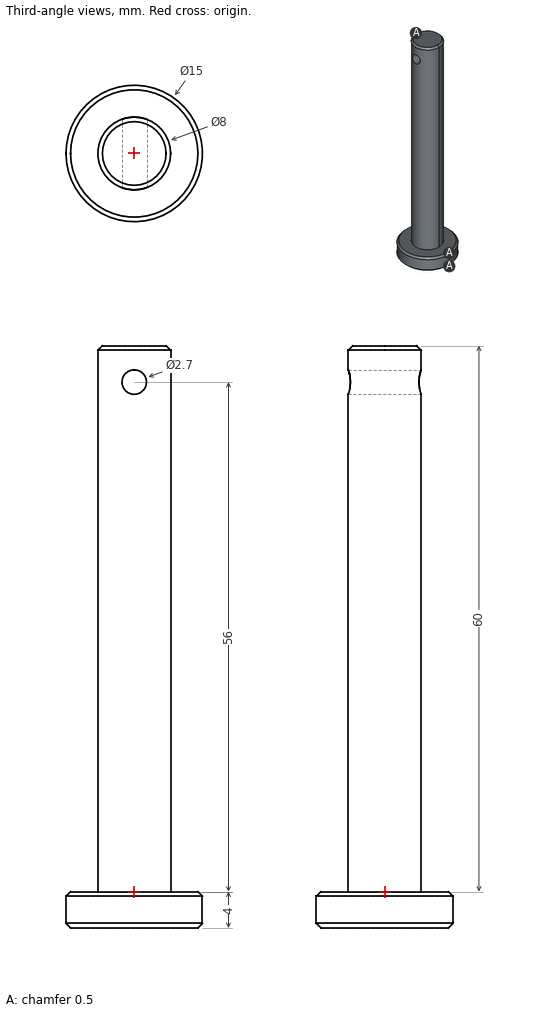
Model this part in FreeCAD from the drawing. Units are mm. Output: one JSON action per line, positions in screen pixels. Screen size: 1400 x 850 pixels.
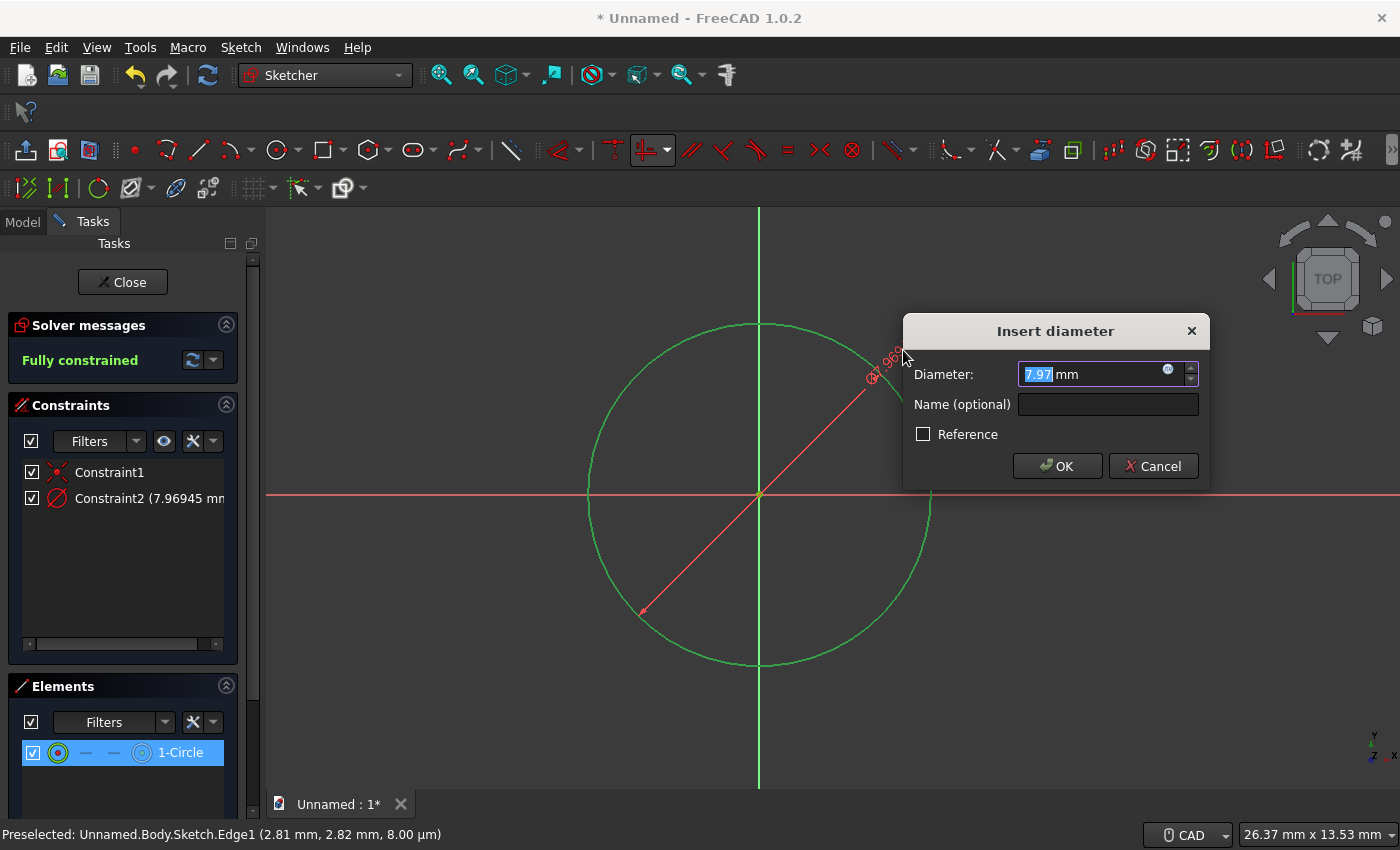
{"action": "type", "text": "8"}
{"action": "key", "text": "Return"}
{"action": "key", "text": "Escape"}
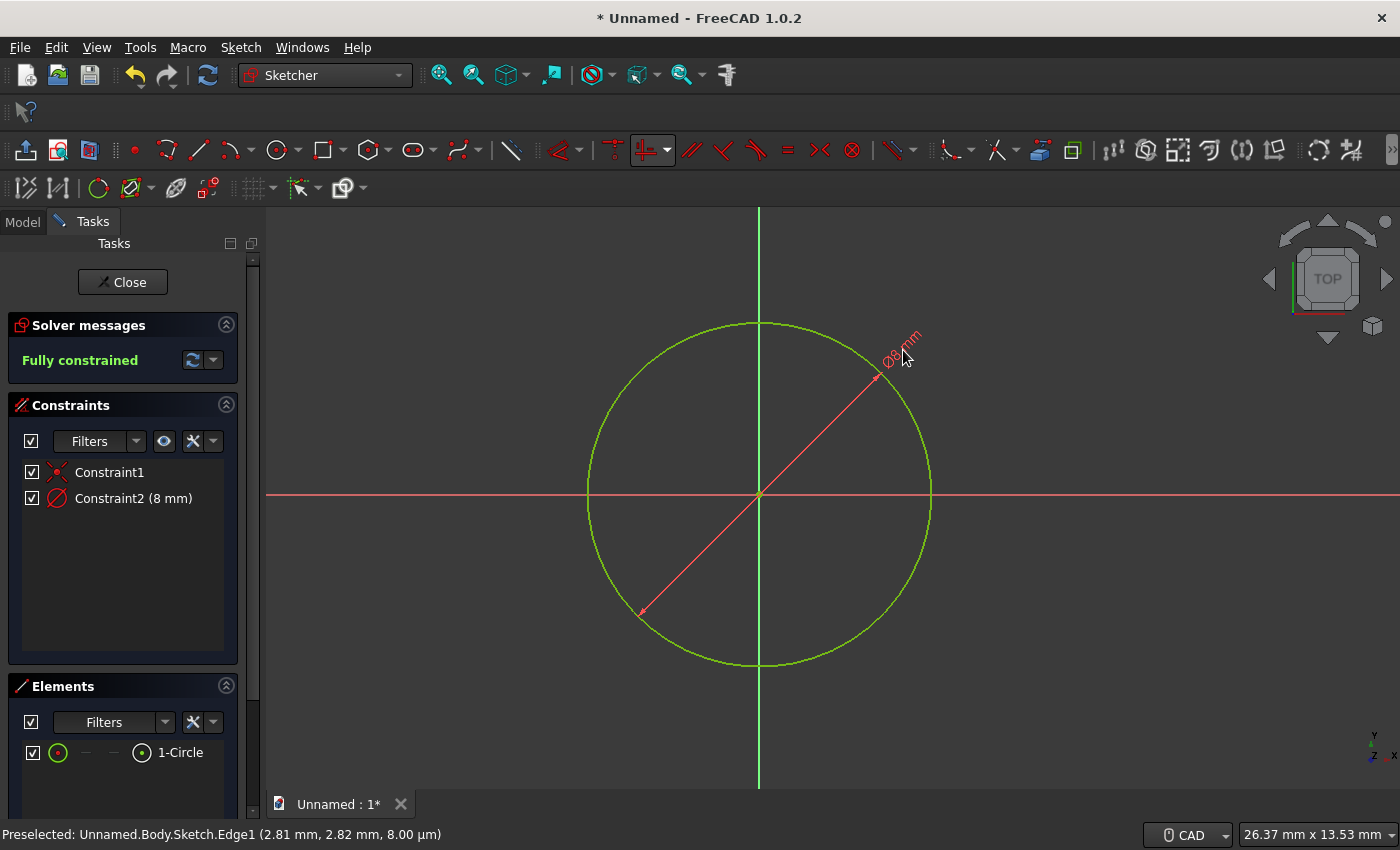
{"action": "left_click", "coordinate": [123, 282]}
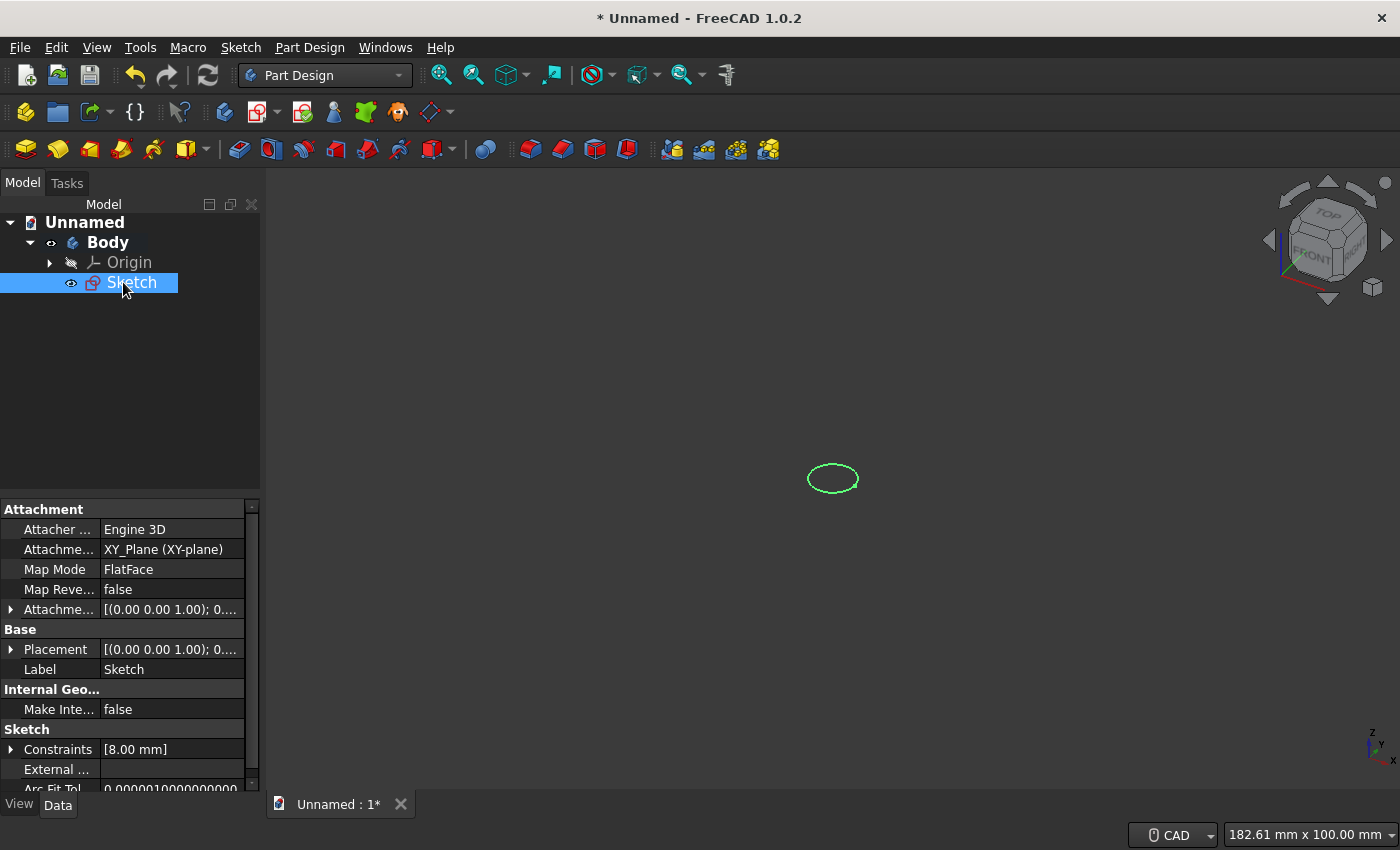
{"action": "left_click", "coordinate": [26, 150]}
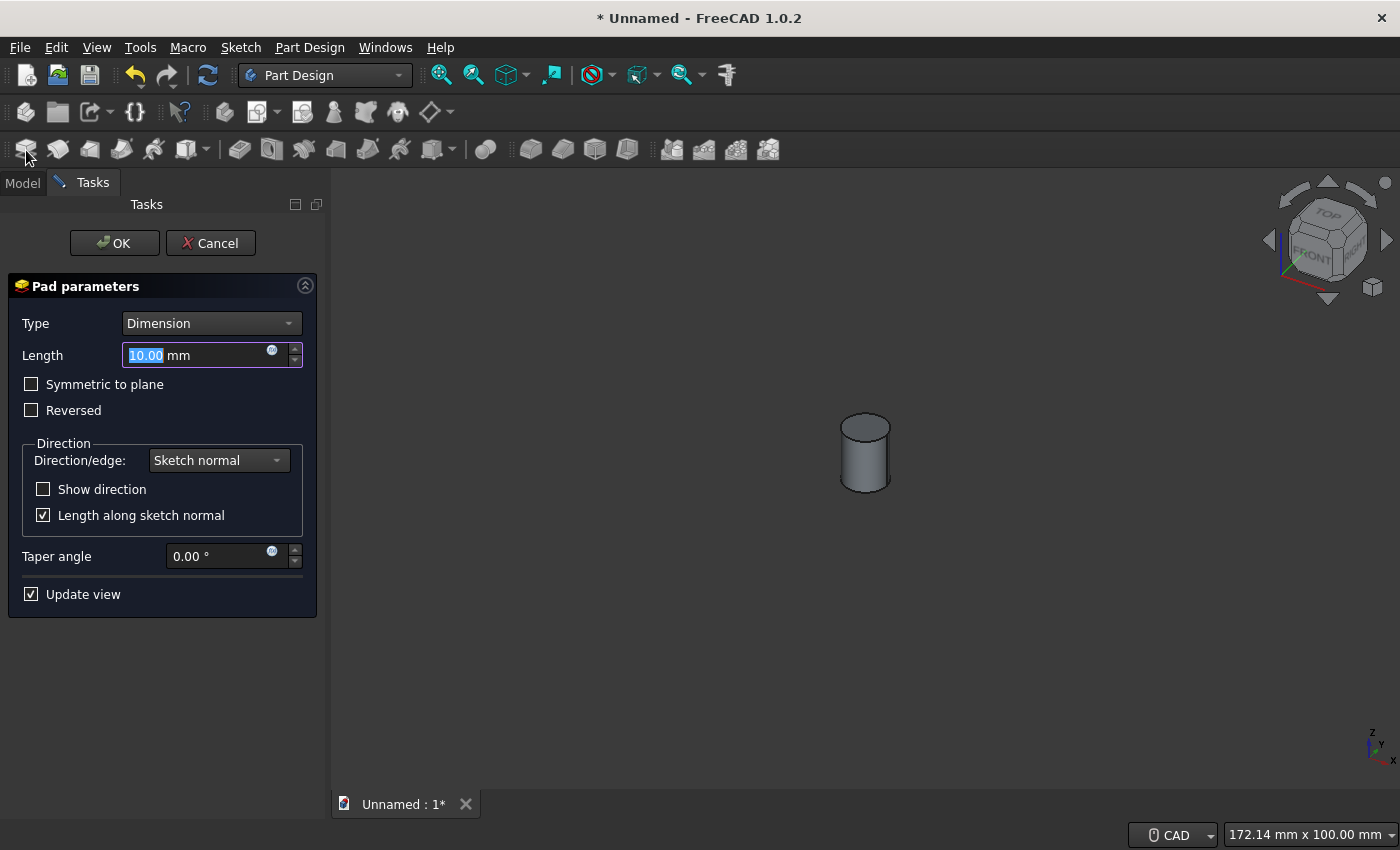
{"action": "type", "text": "60"}
{"action": "key", "text": "Tab"}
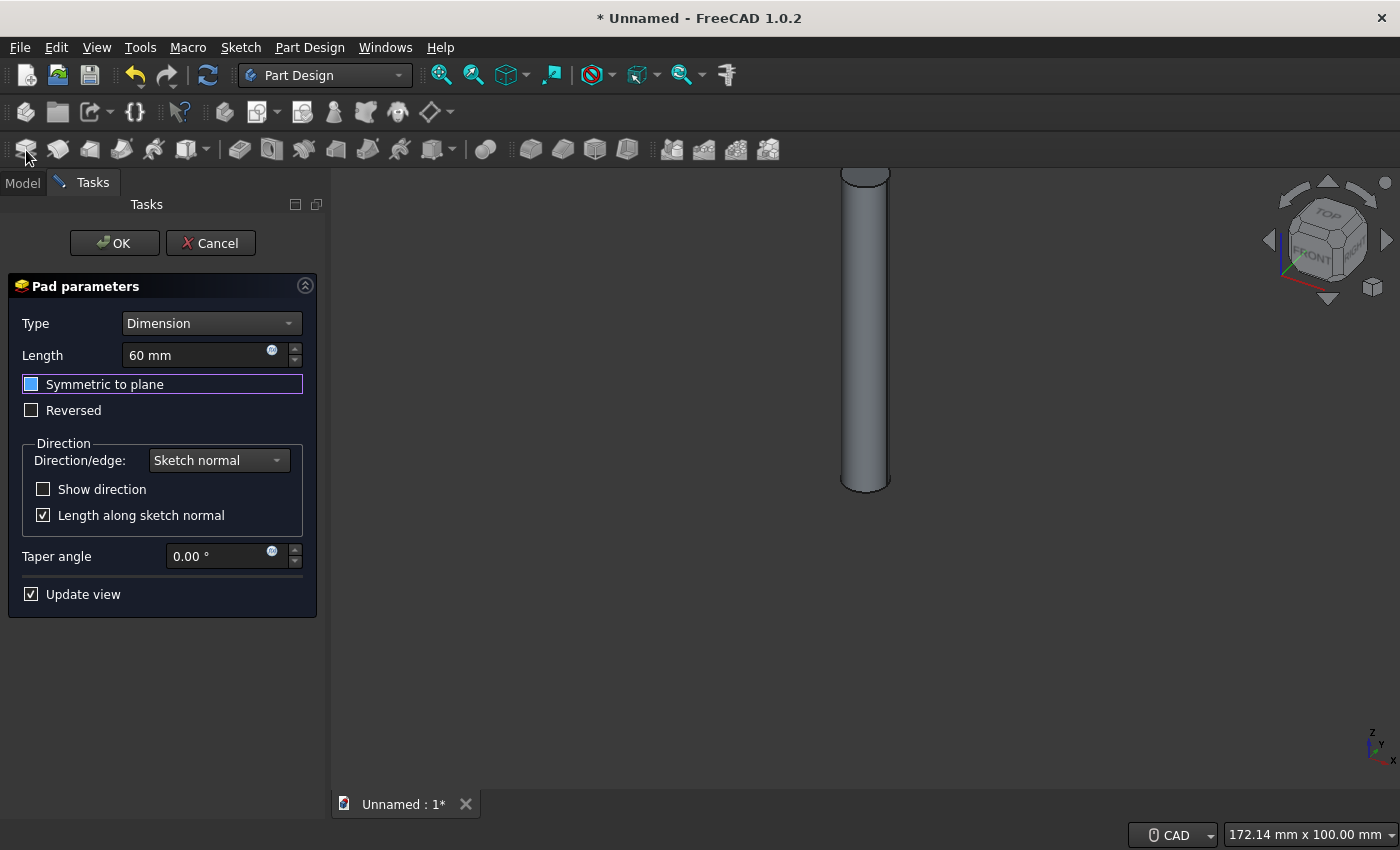
{"action": "left_click", "coordinate": [115, 243]}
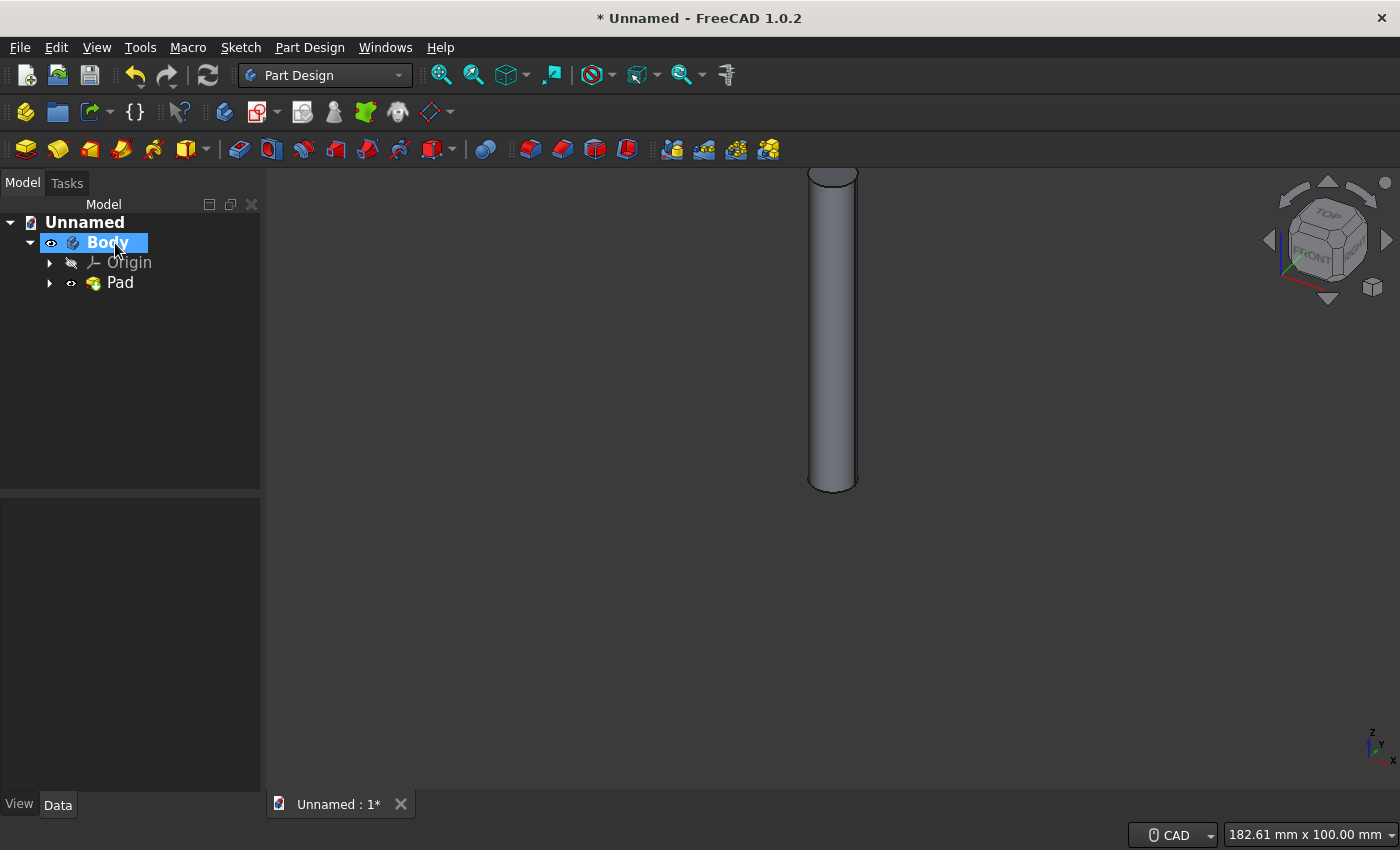
{"action": "left_click", "coordinate": [442, 76]}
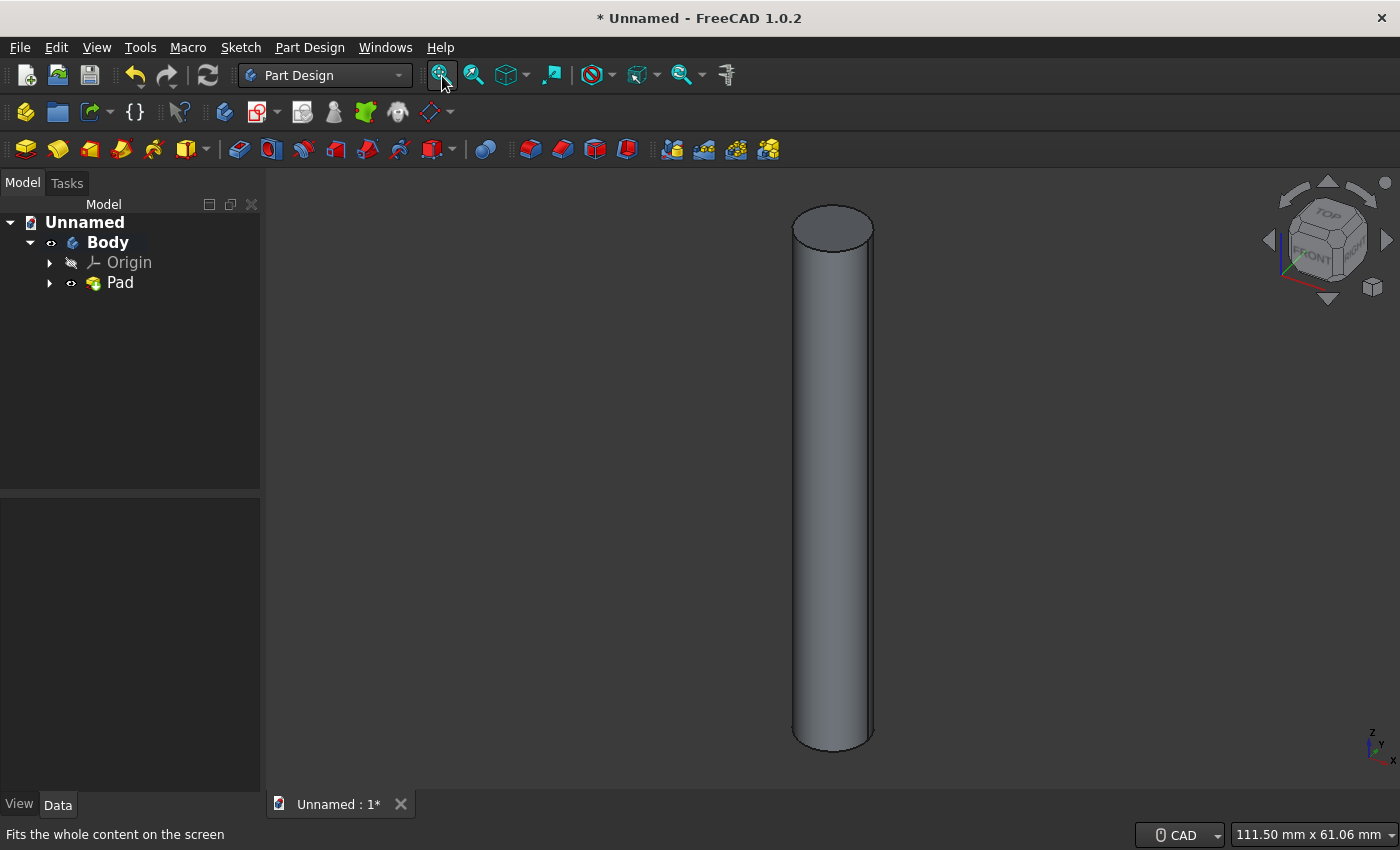
{"action": "left_click", "coordinate": [258, 112]}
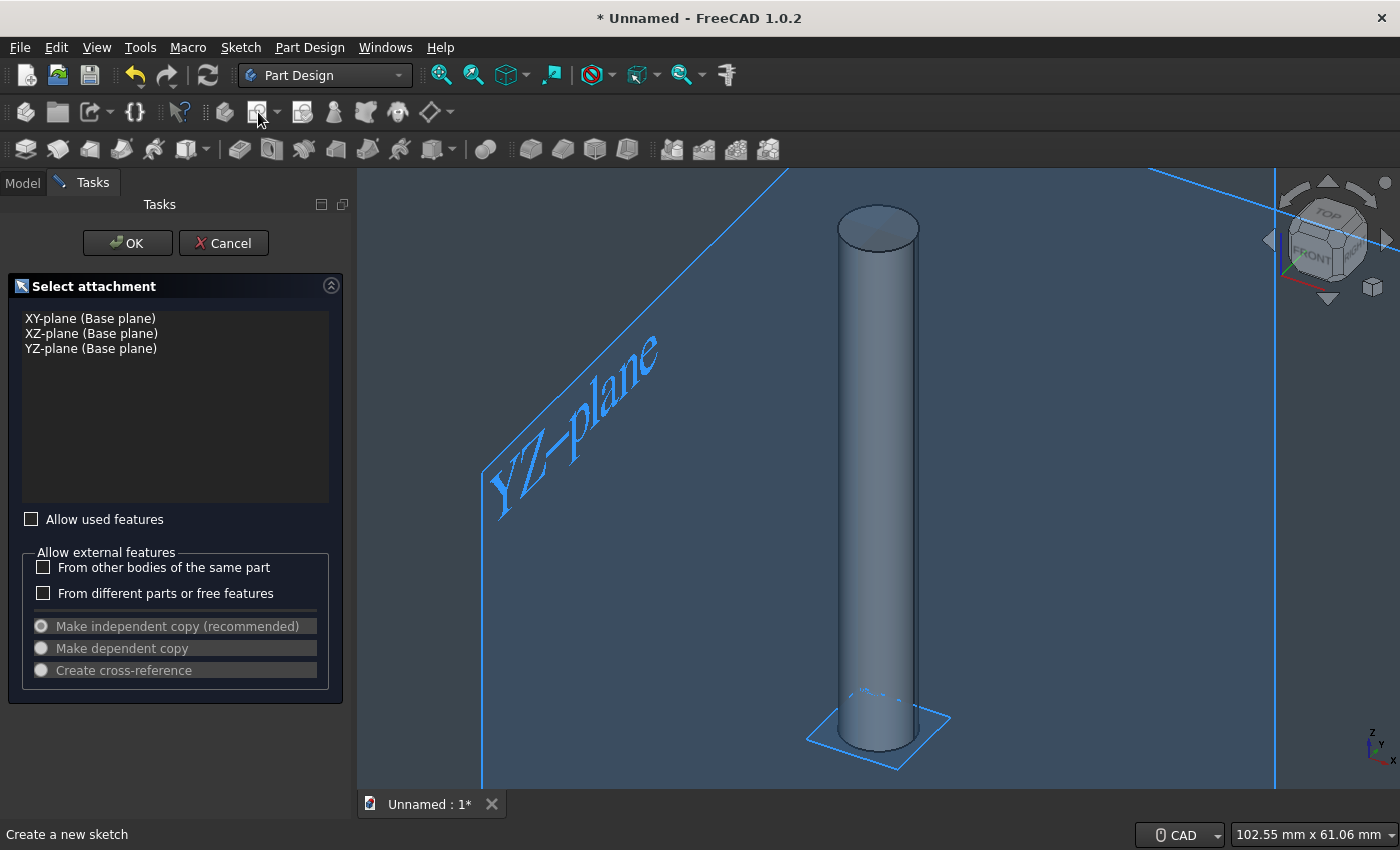
{"action": "left_click", "coordinate": [82, 318]}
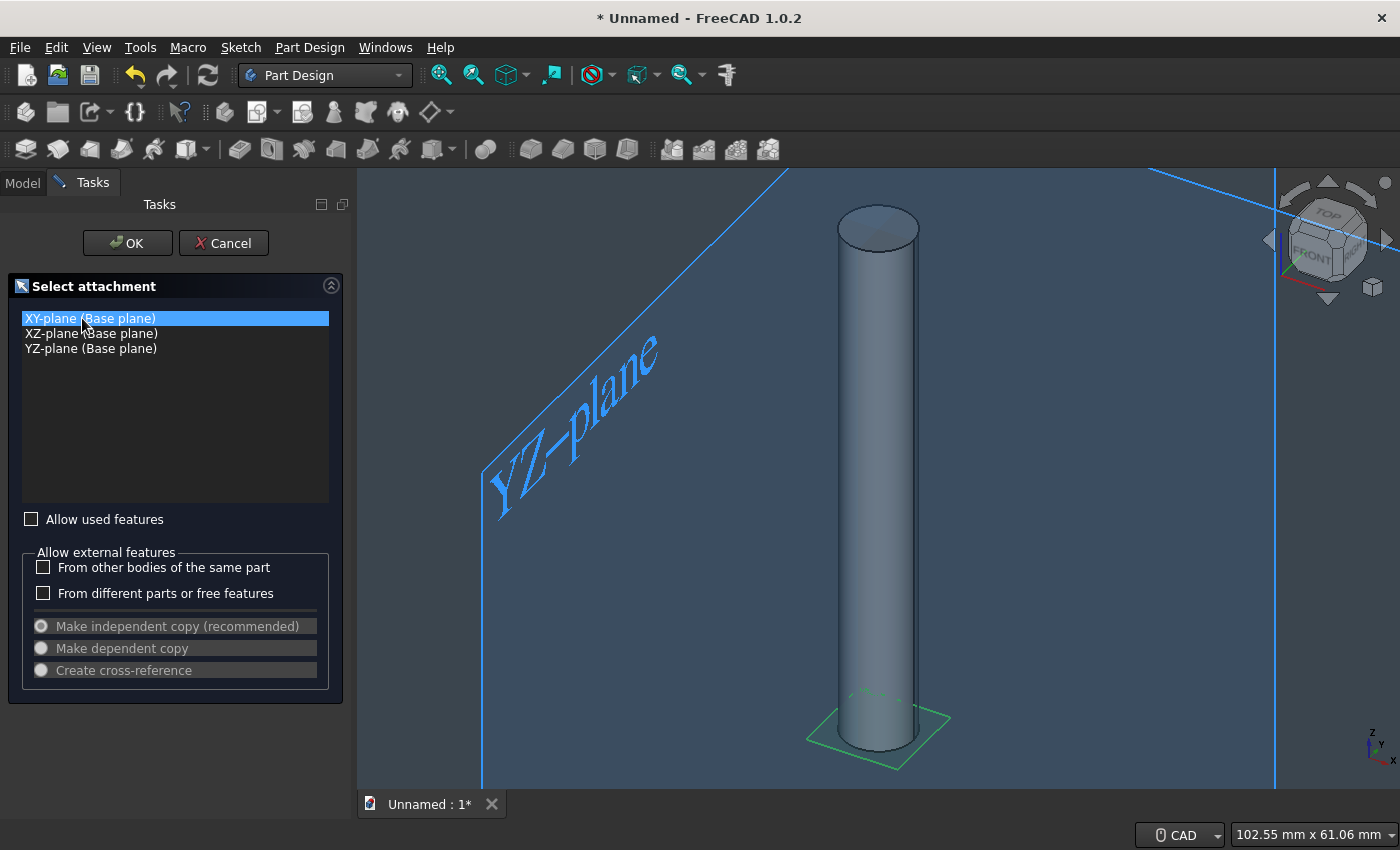
{"action": "left_click", "coordinate": [128, 243]}